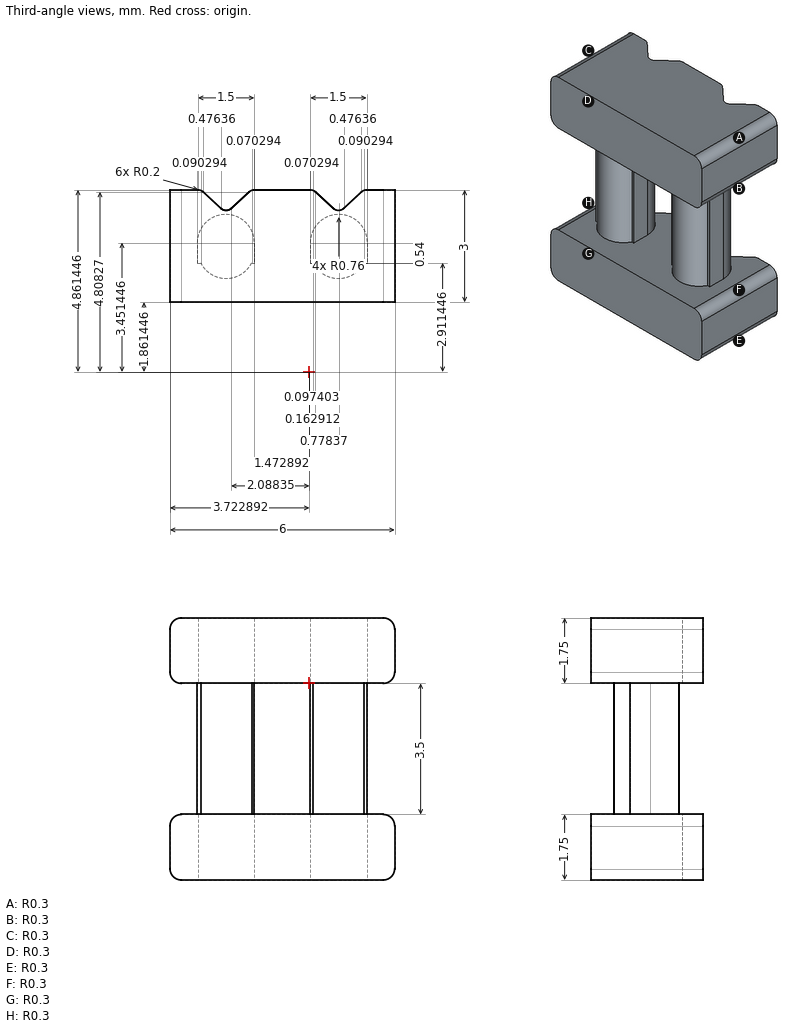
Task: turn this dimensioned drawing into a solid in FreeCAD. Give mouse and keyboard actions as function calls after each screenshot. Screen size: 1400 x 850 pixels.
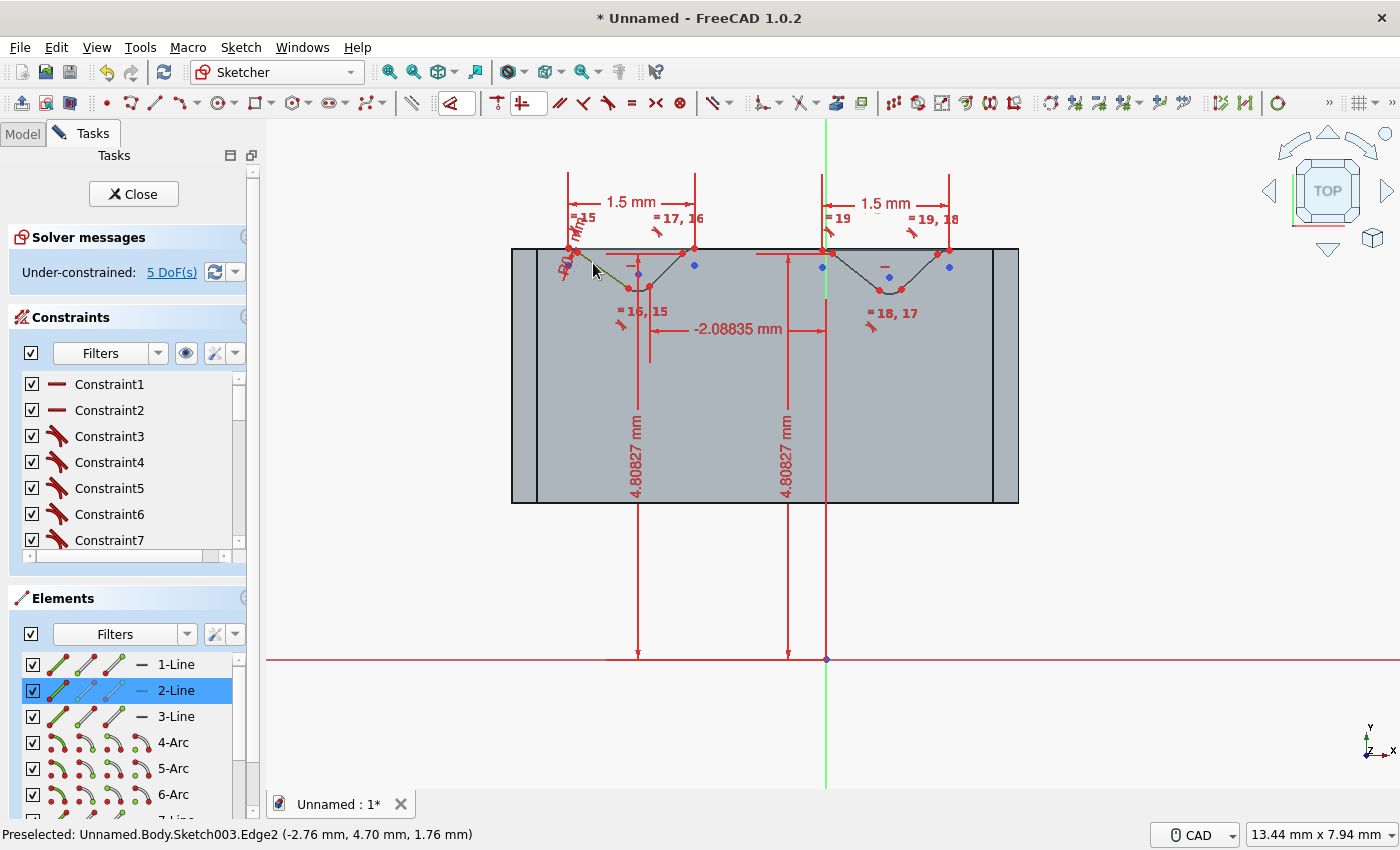
click(470, 104)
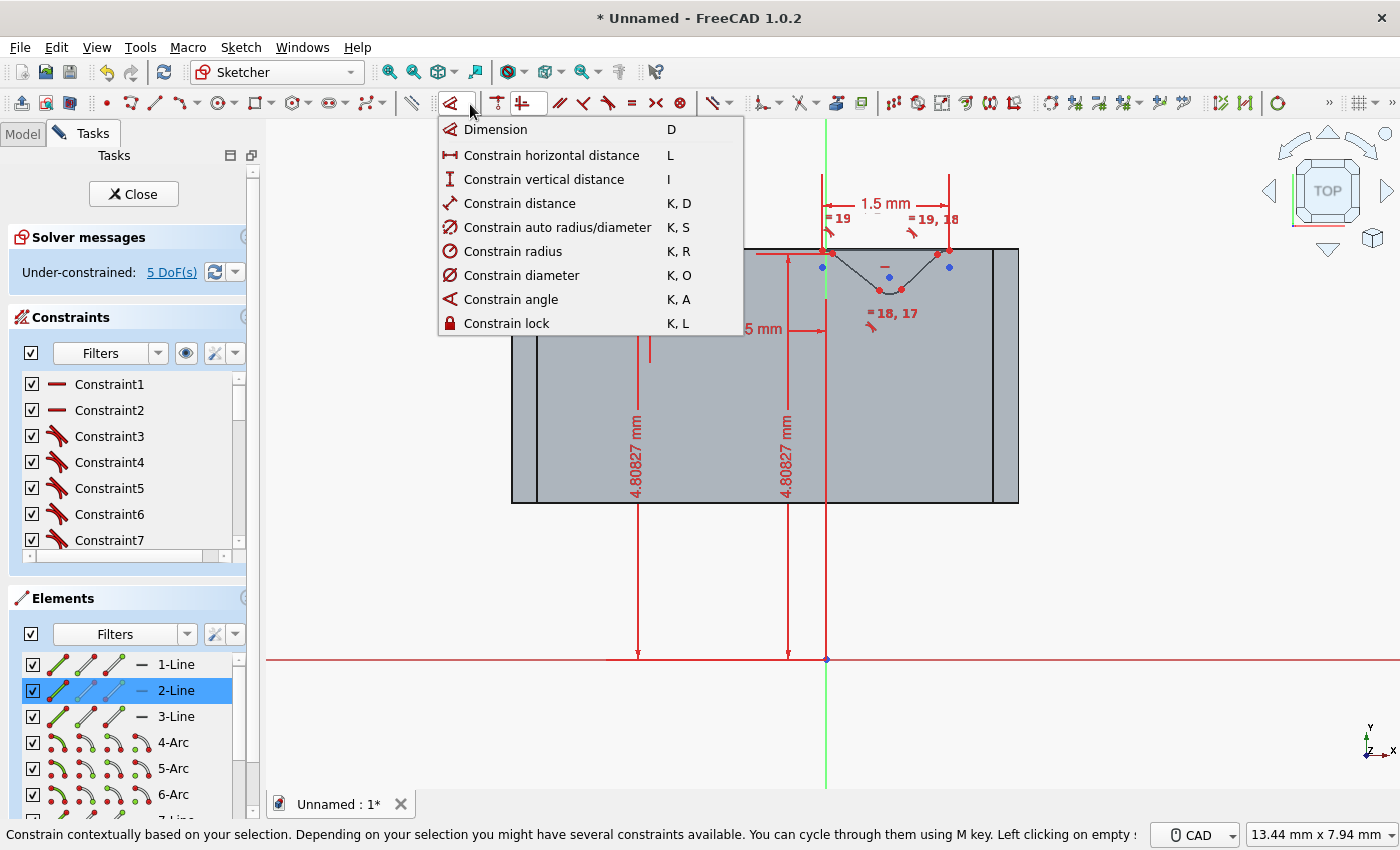
click(591, 155)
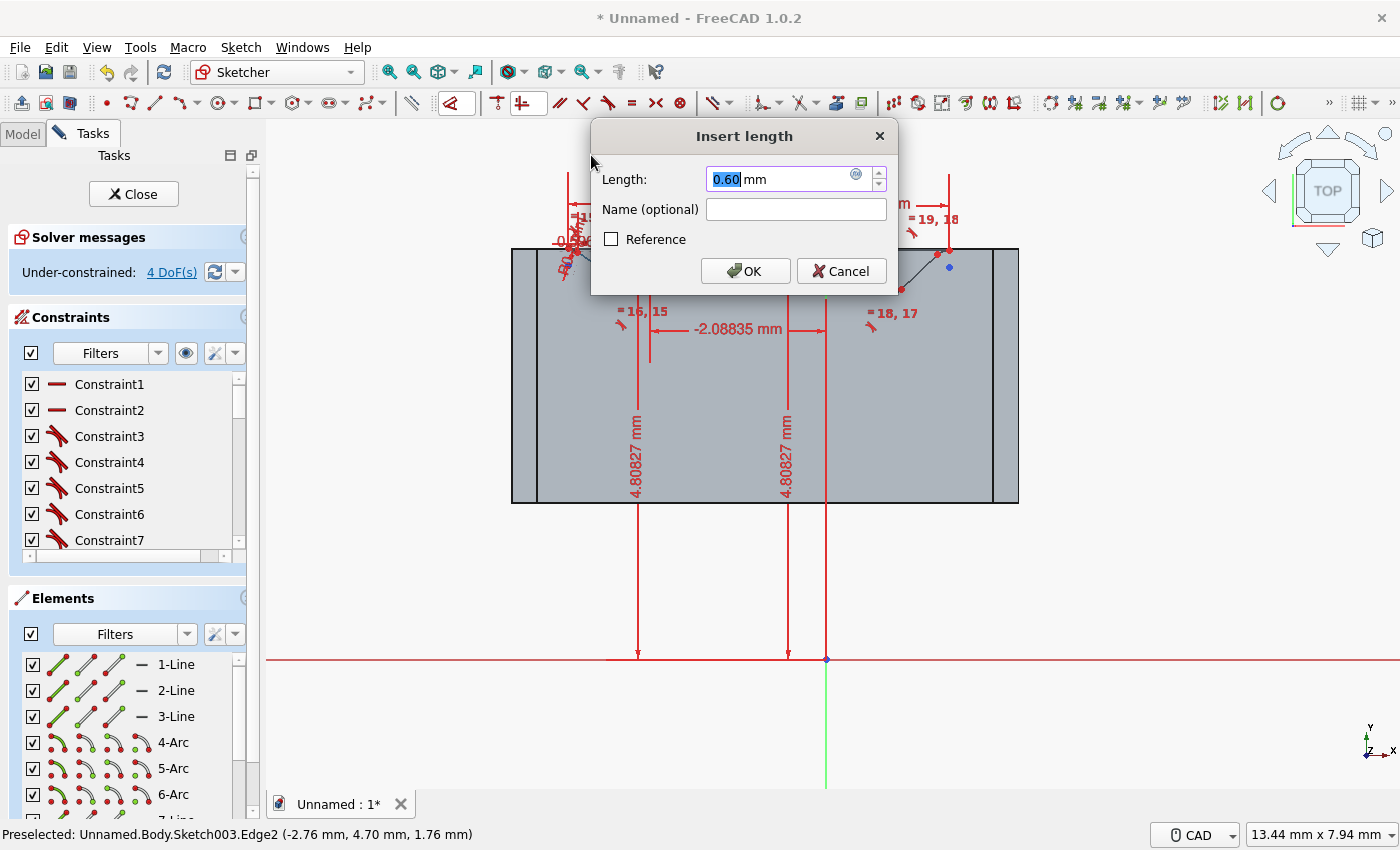
text(0.47636)
key(Return)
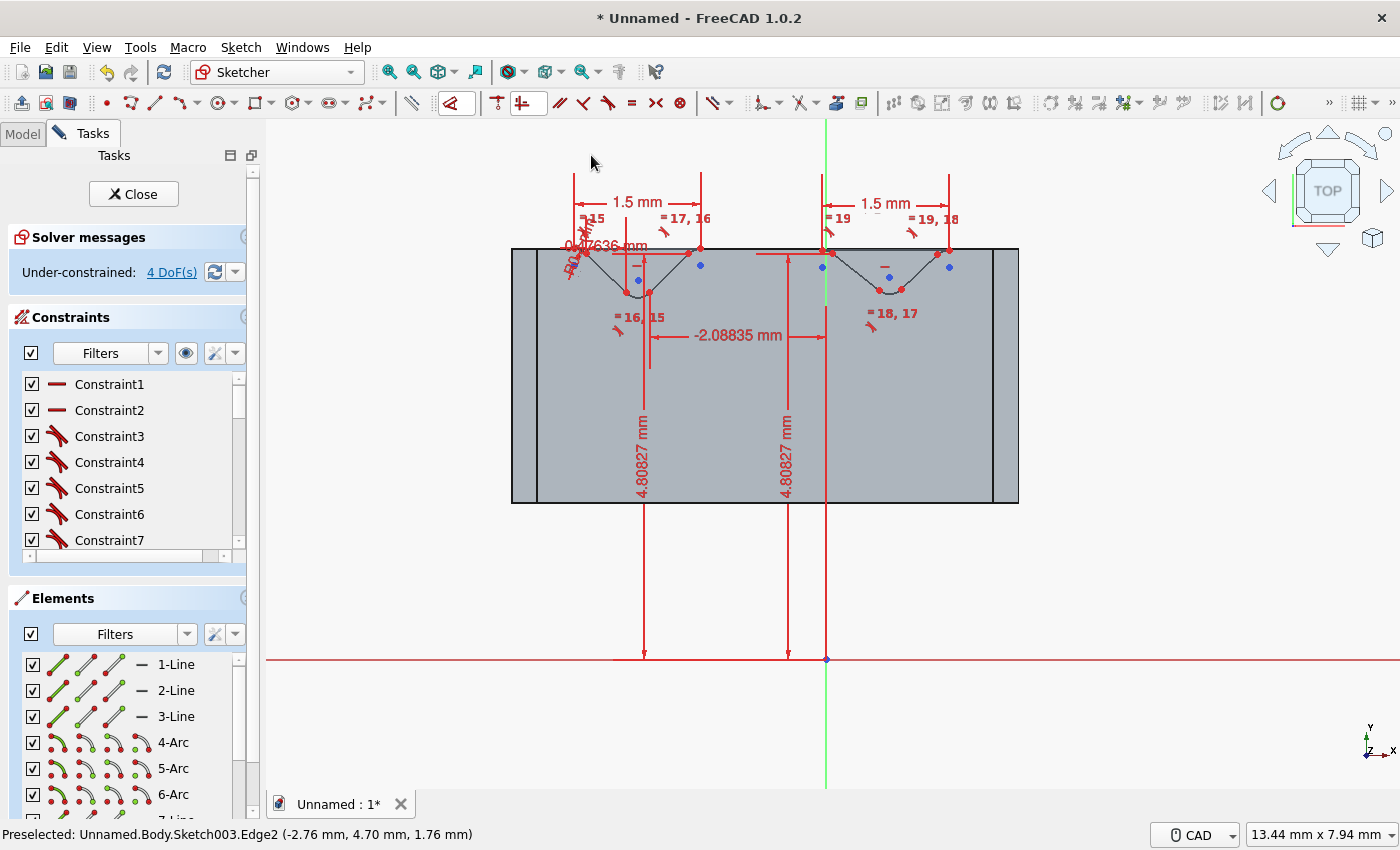
click(912, 279)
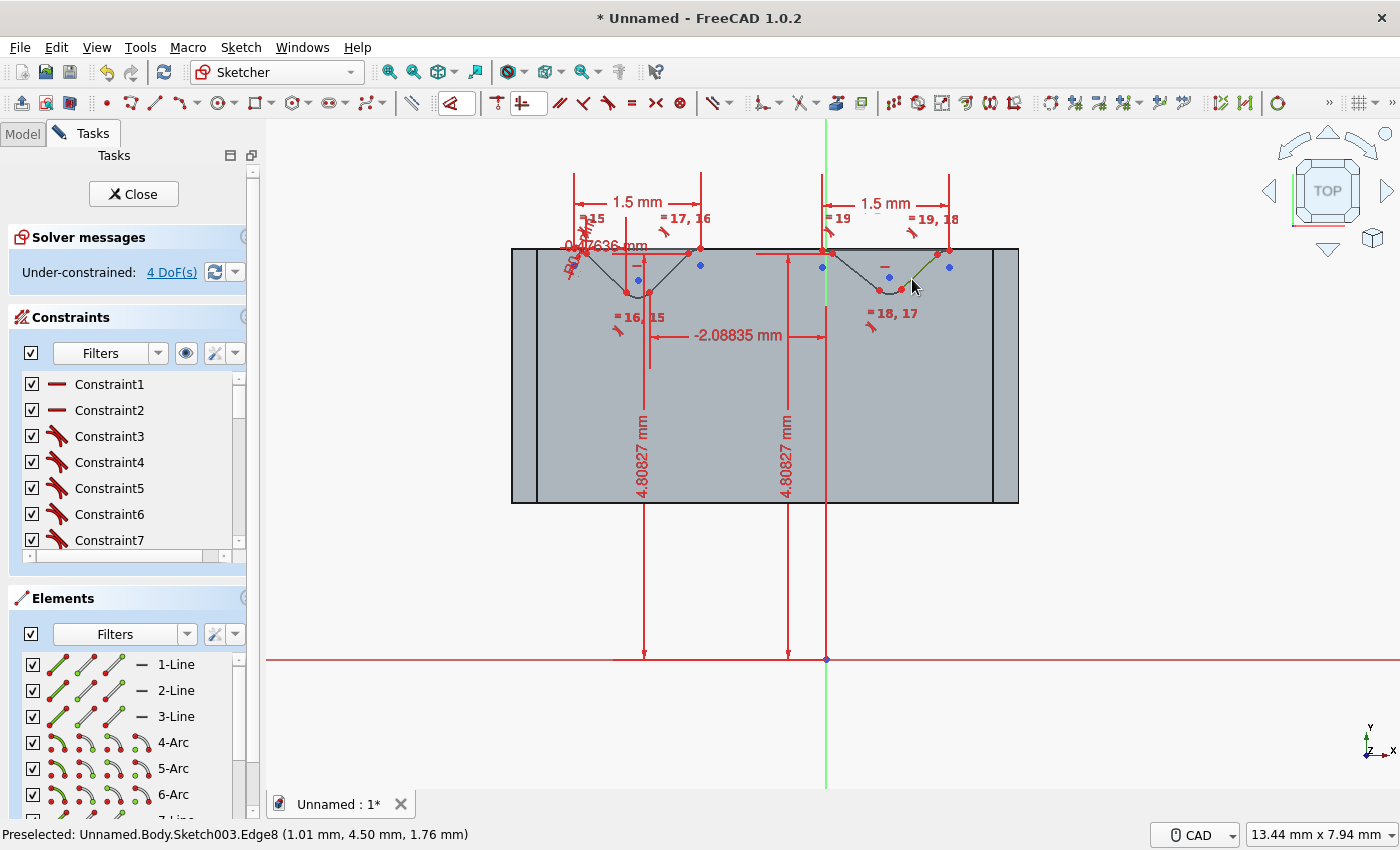
click(470, 104)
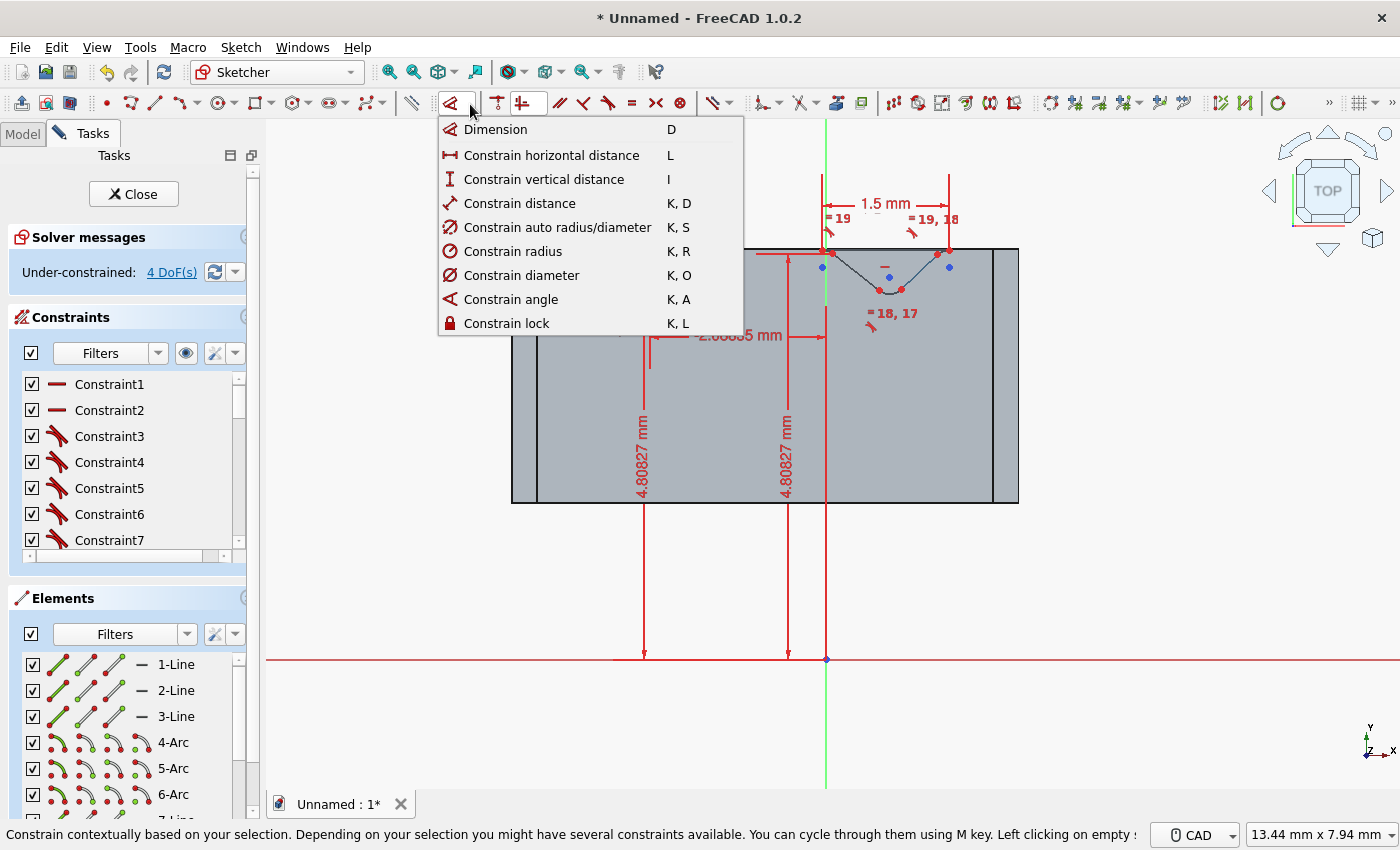
click(591, 155)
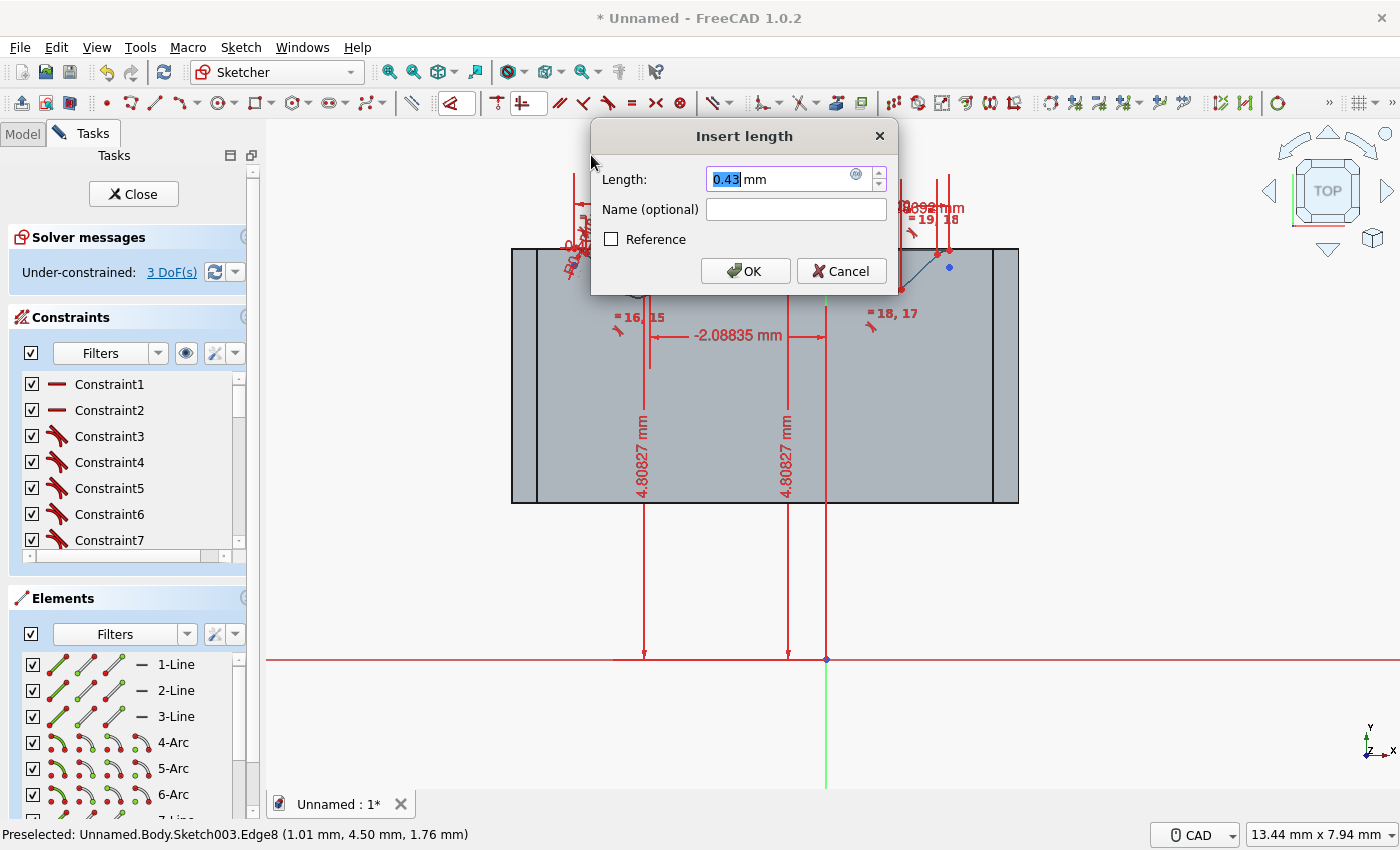
text(0.47636)
key(Return)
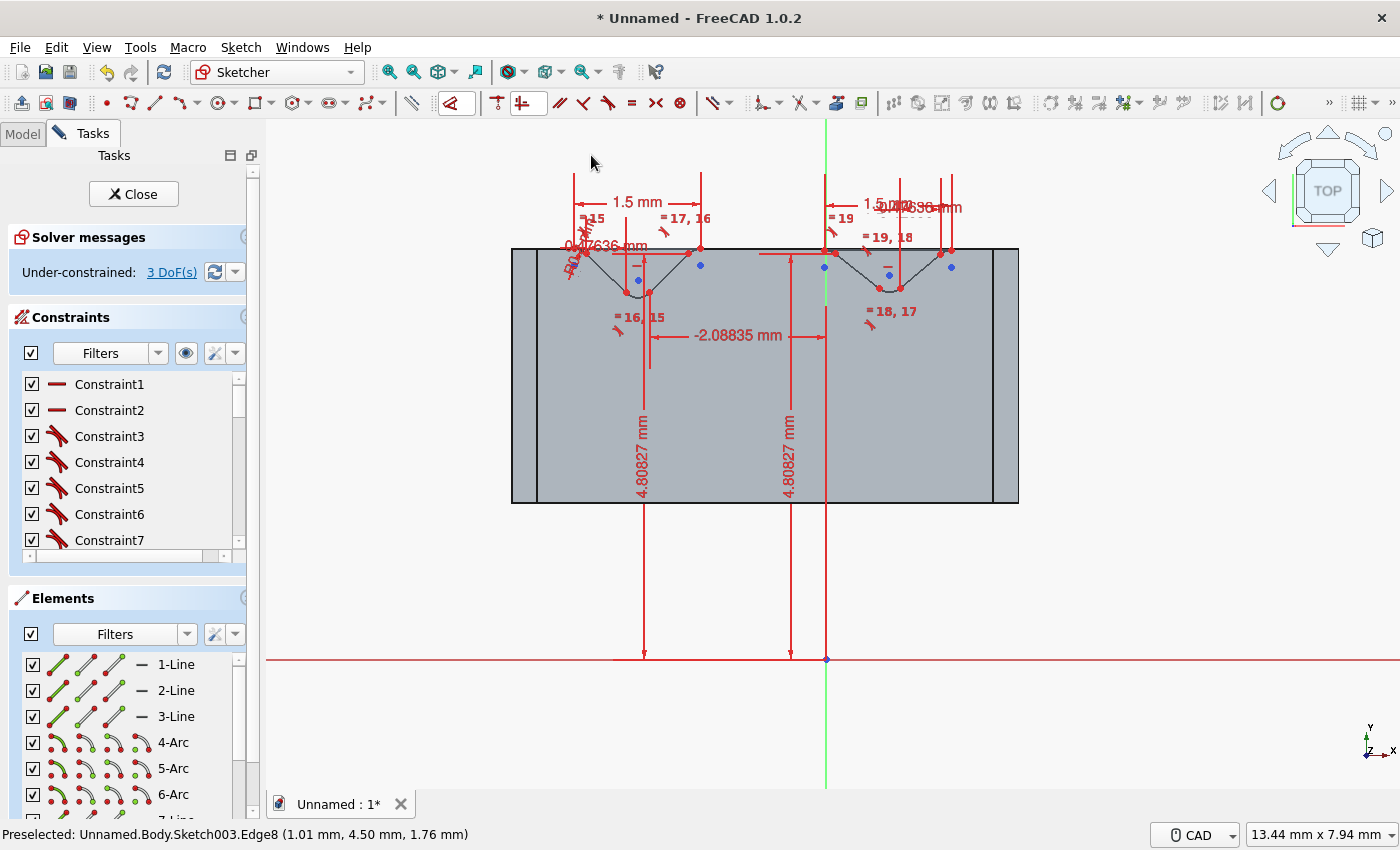
click(890, 275)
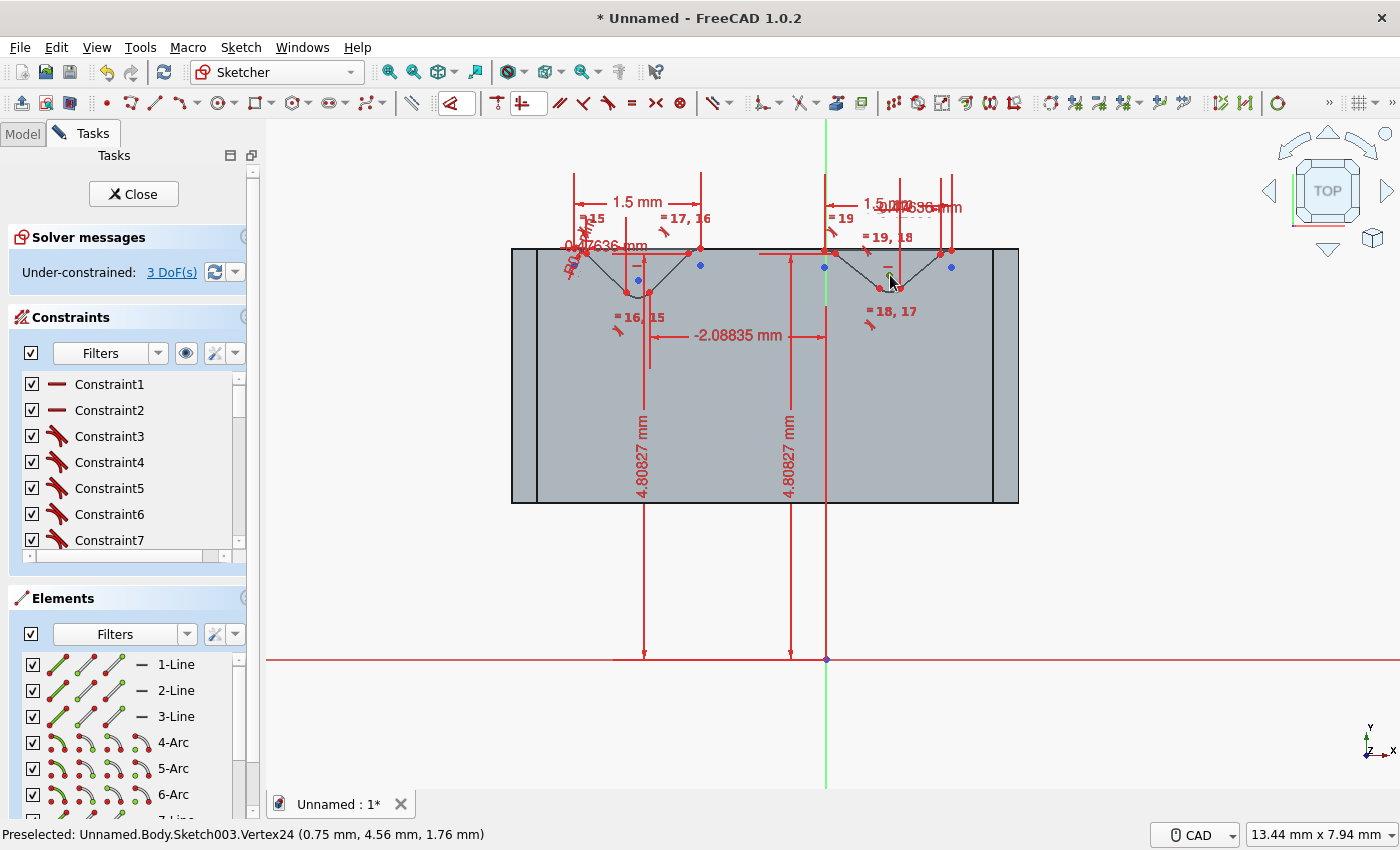
click(470, 104)